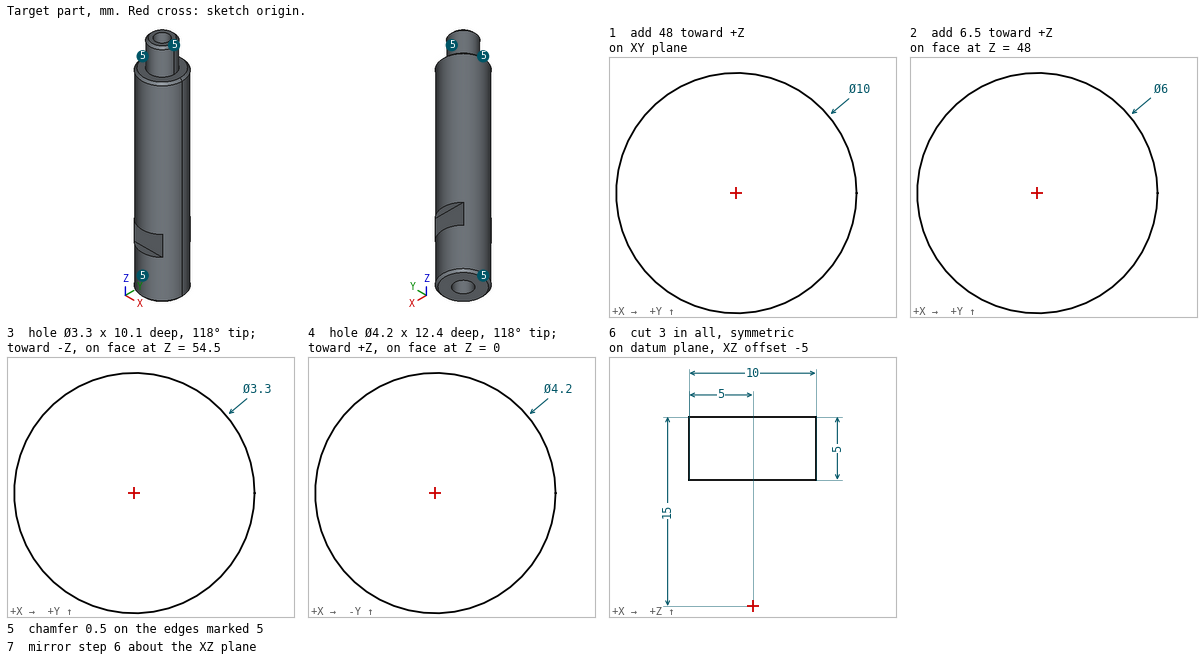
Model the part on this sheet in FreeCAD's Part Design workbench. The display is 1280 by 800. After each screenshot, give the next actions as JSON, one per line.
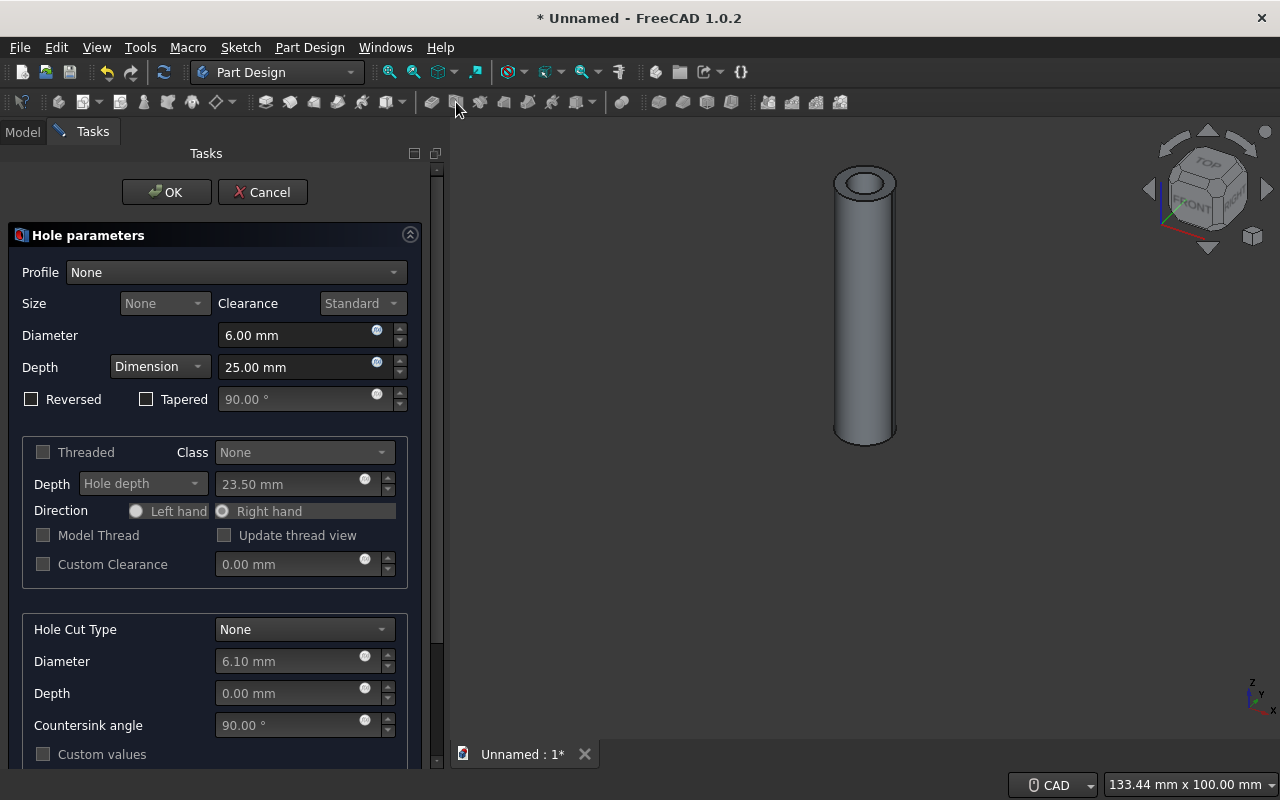
{"action": "triple_click", "coordinate": [305, 335]}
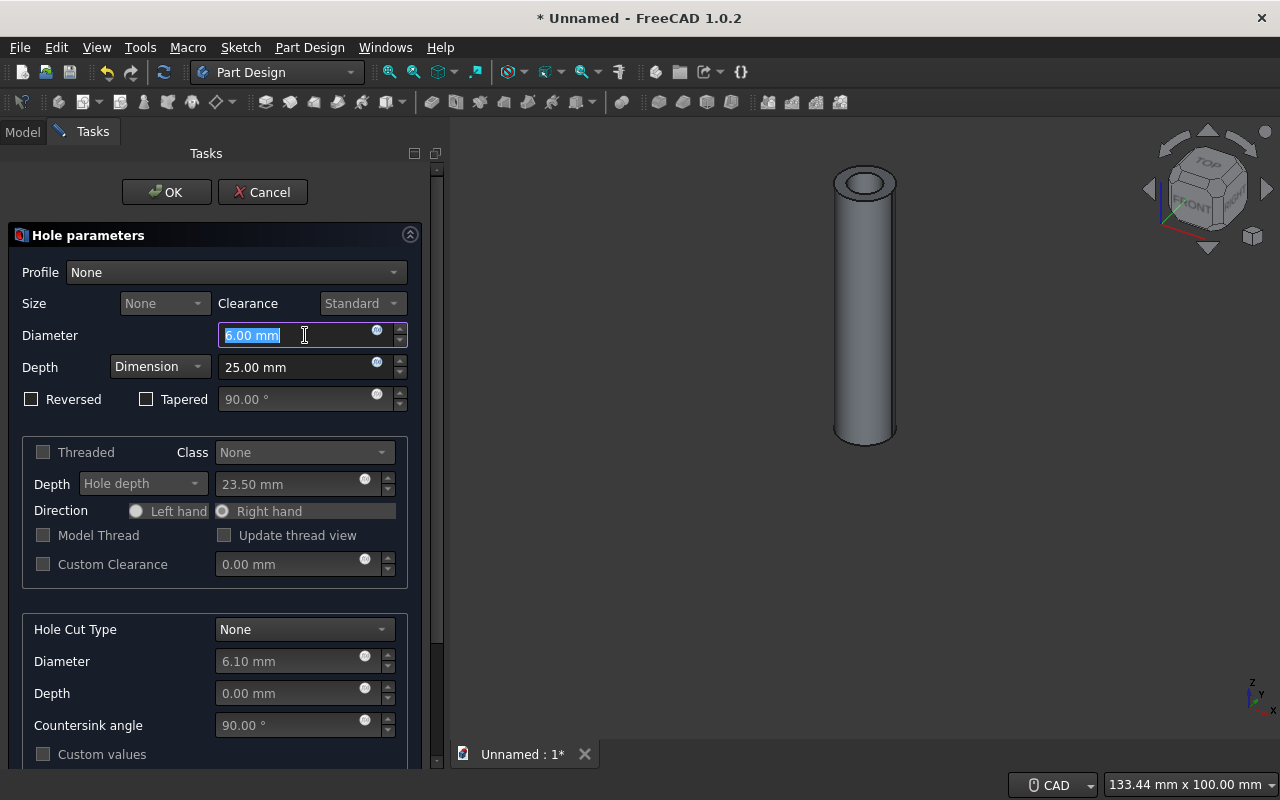
{"action": "type", "text": "3.3"}
{"action": "key", "text": "Tab"}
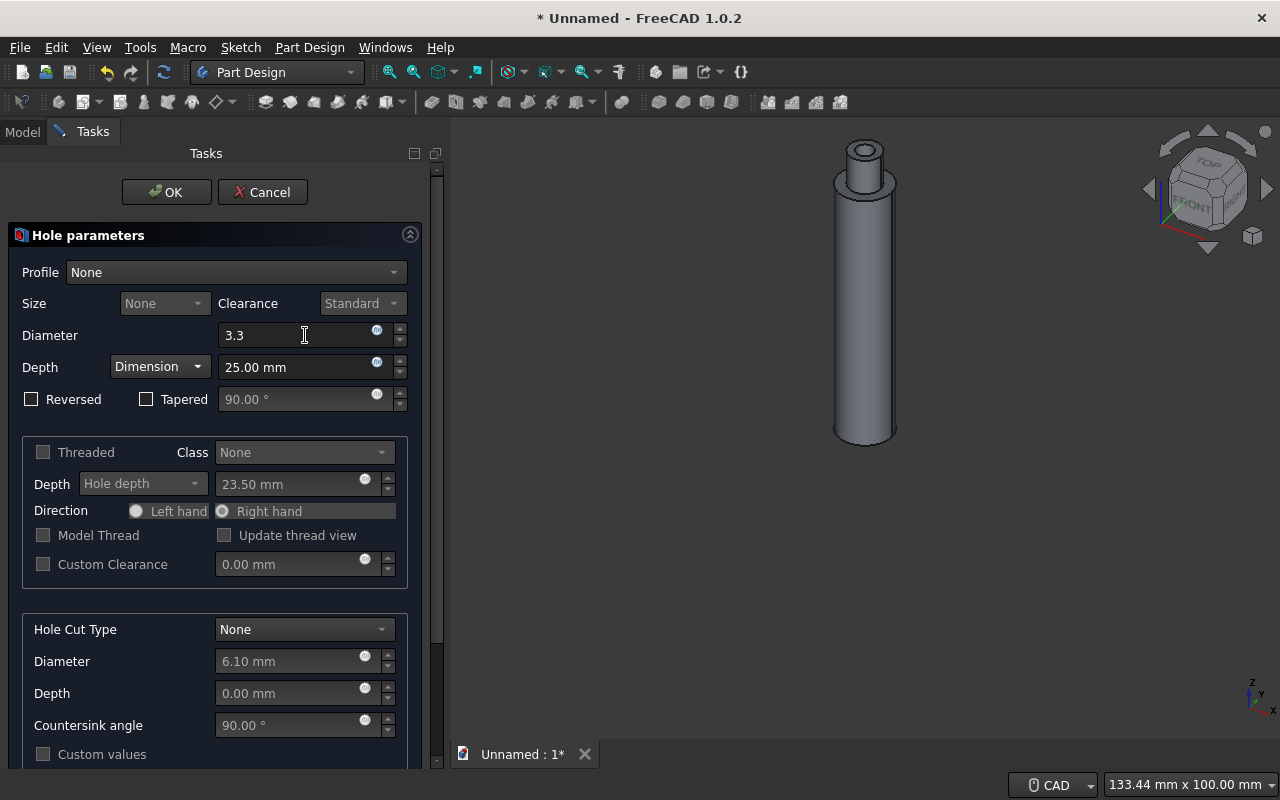
{"action": "triple_click", "coordinate": [305, 367]}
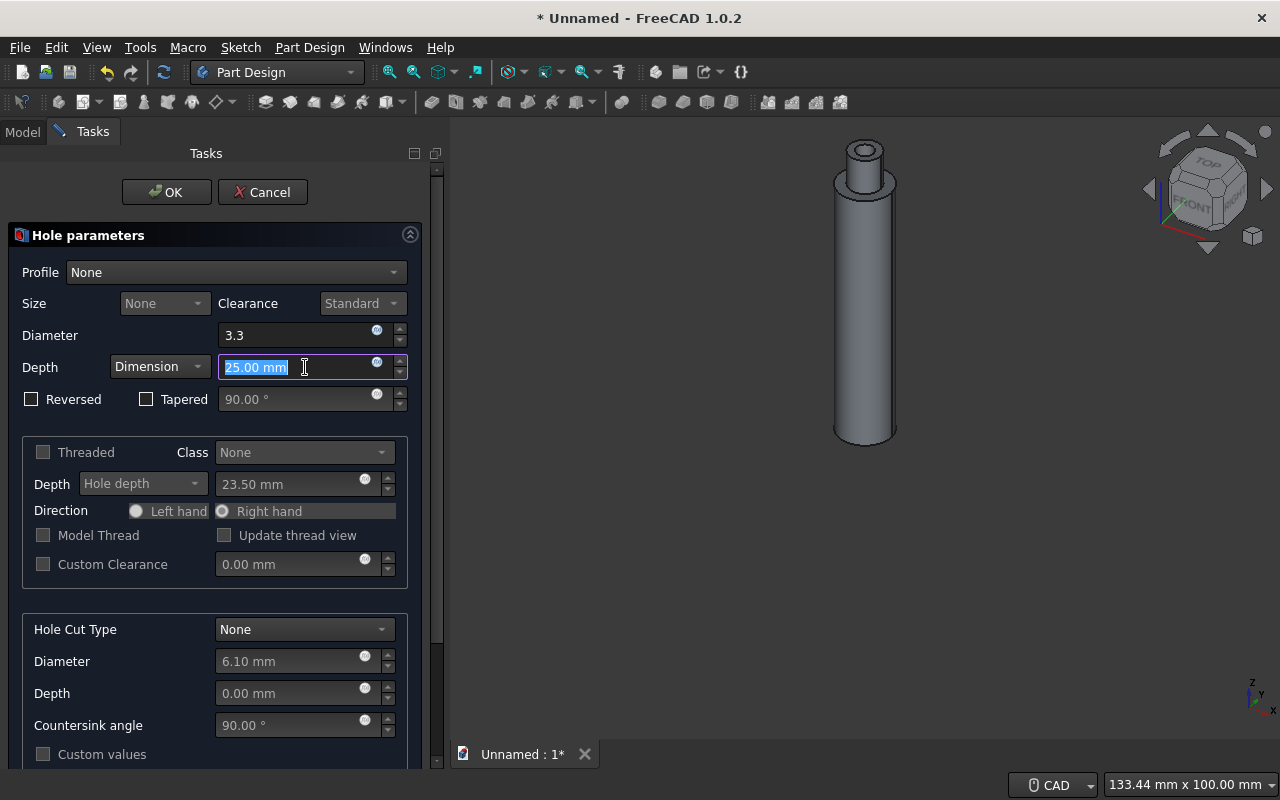
{"action": "type", "text": "10.1"}
{"action": "key", "text": "Tab"}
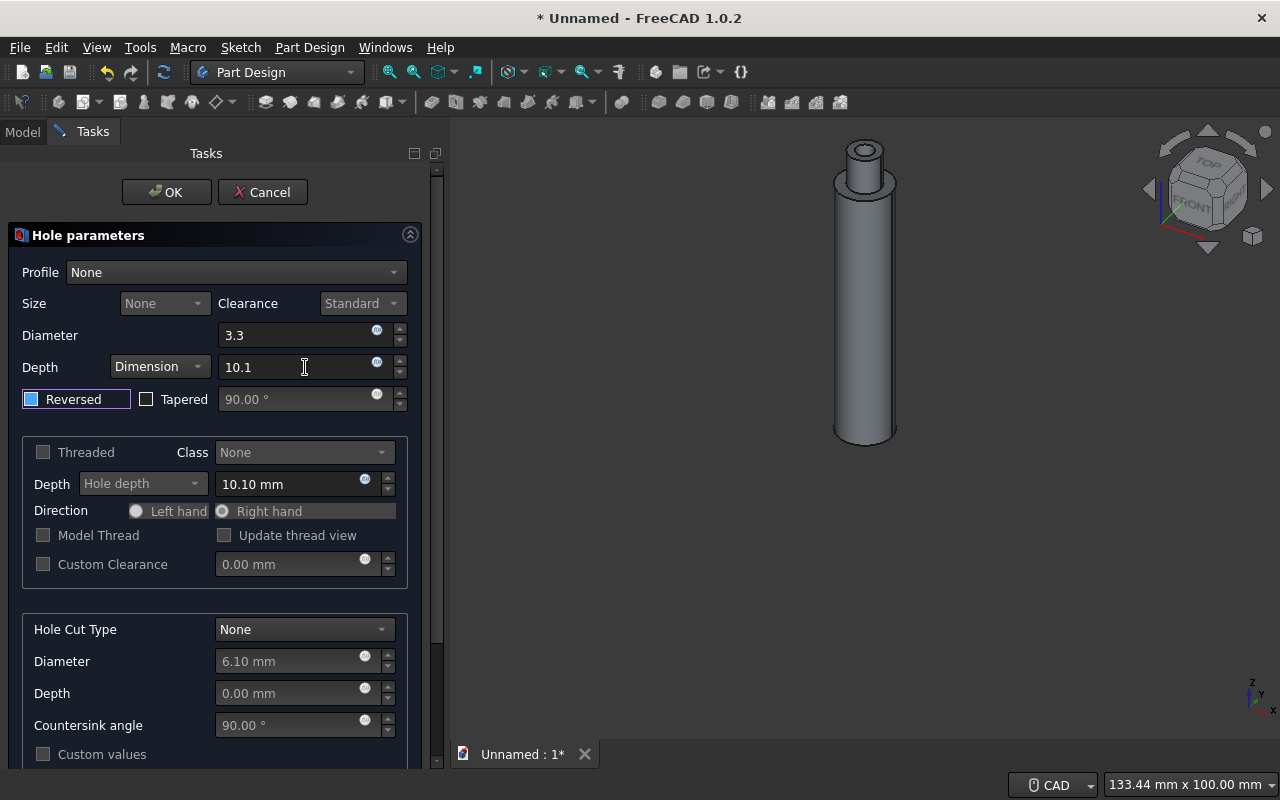
{"action": "left_click", "coordinate": [167, 192]}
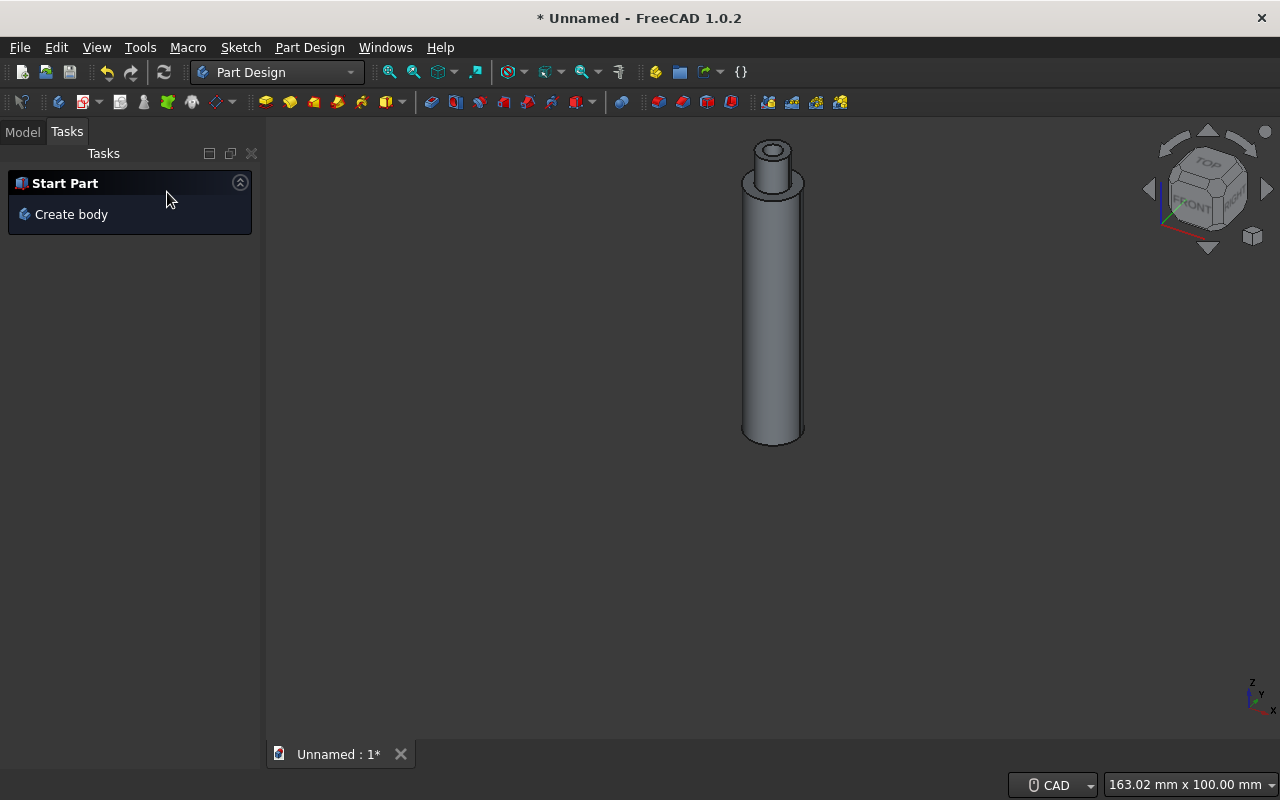
{"action": "key", "text": "5"}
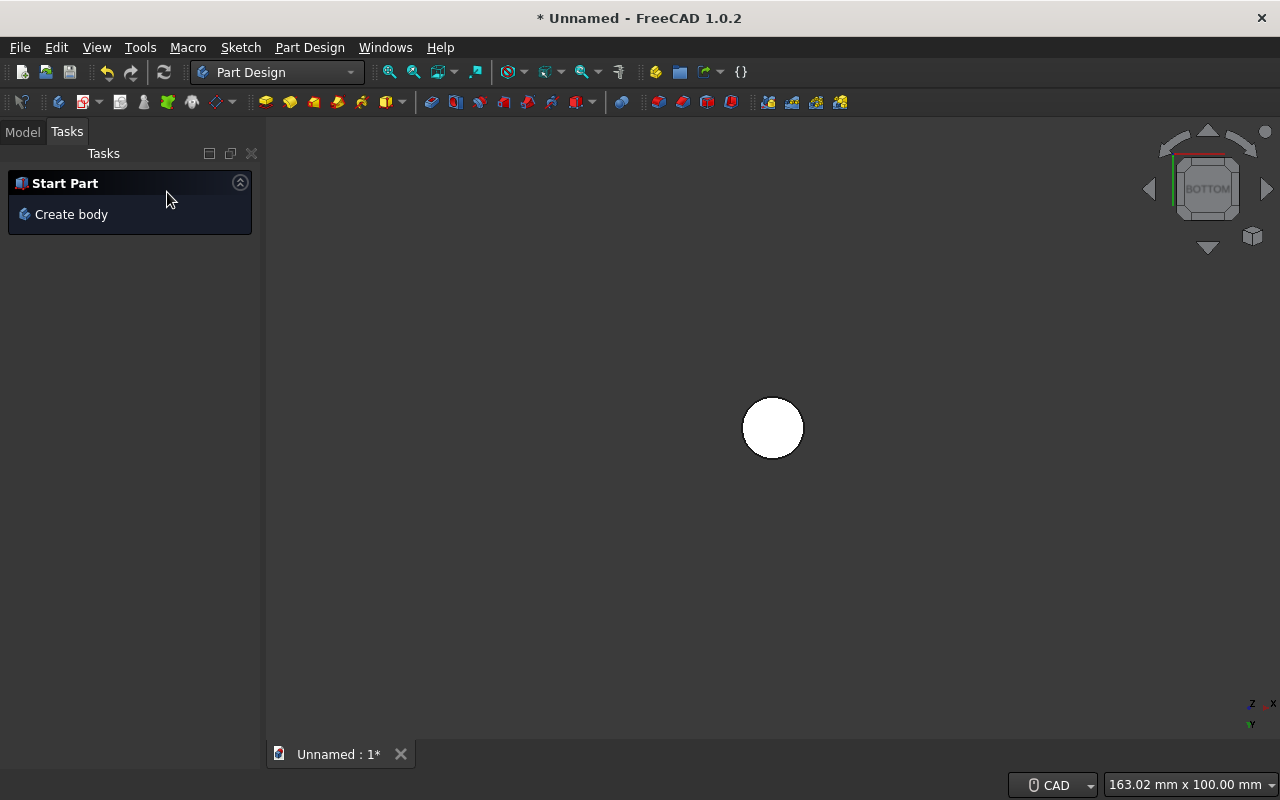
{"action": "left_click", "coordinate": [390, 72]}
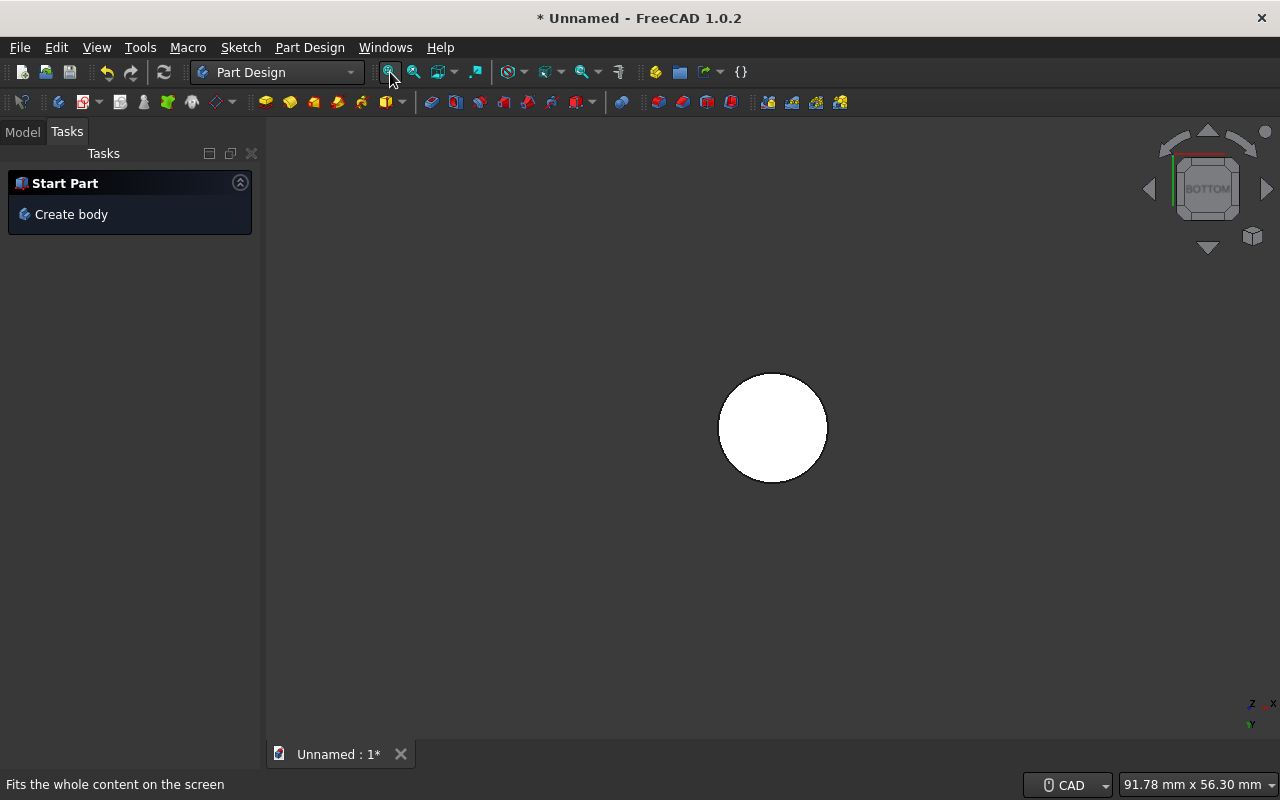
{"action": "left_click", "coordinate": [773, 427]}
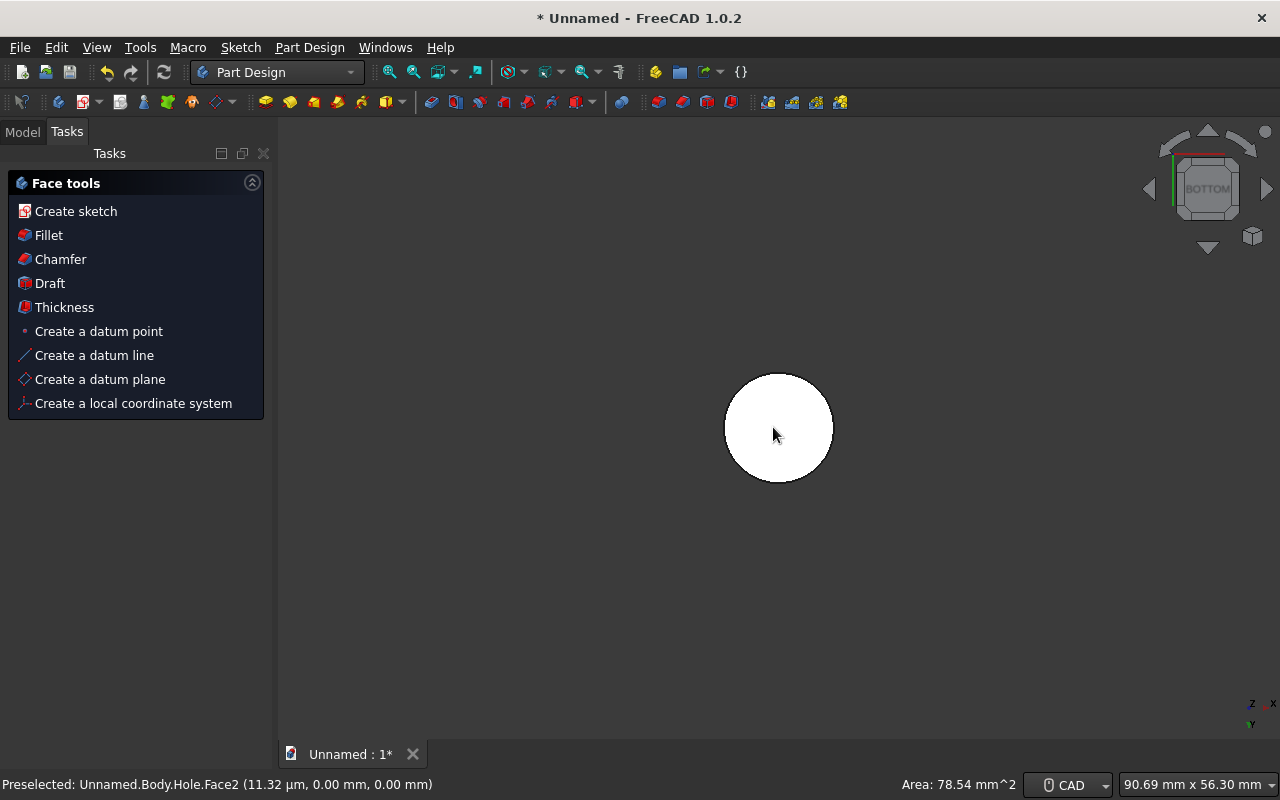
{"action": "left_click", "coordinate": [84, 102]}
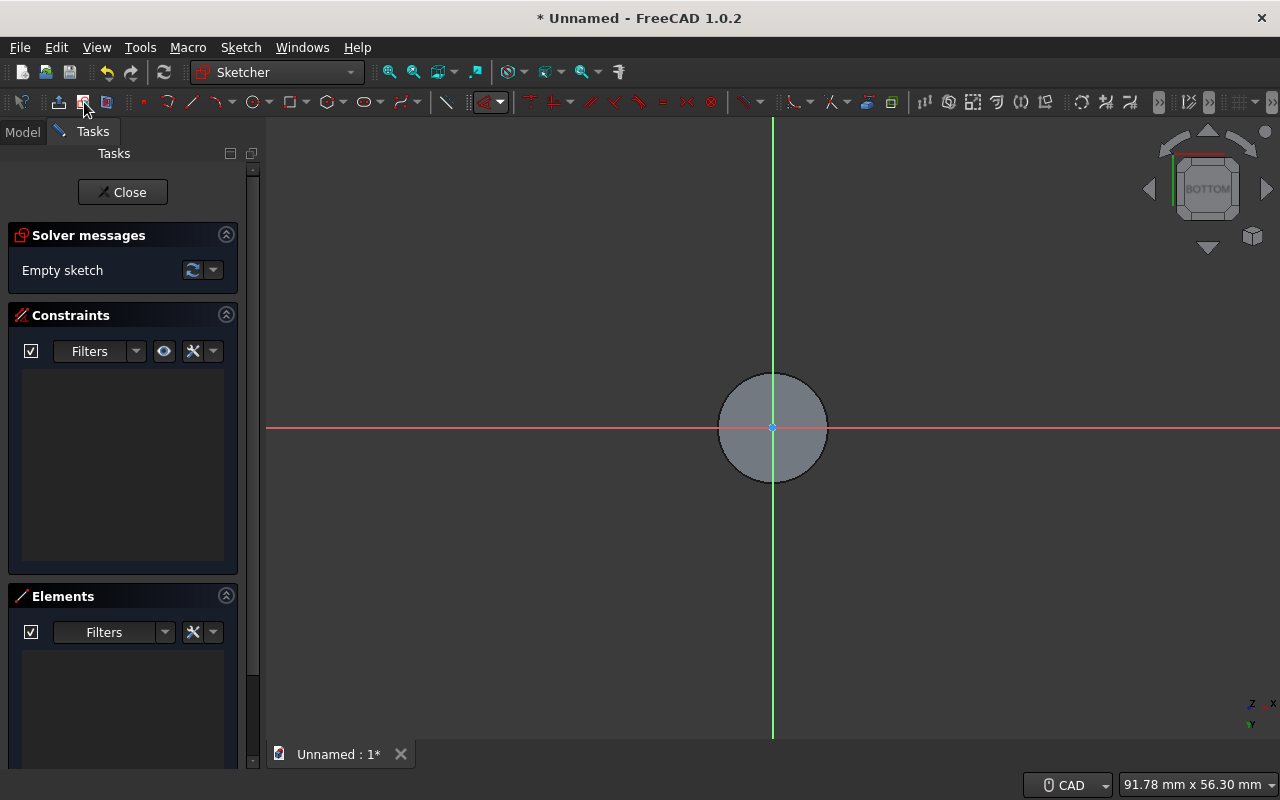
{"action": "scroll", "coordinate": [781, 428], "scroll_direction": "up", "scroll_amount": 11}